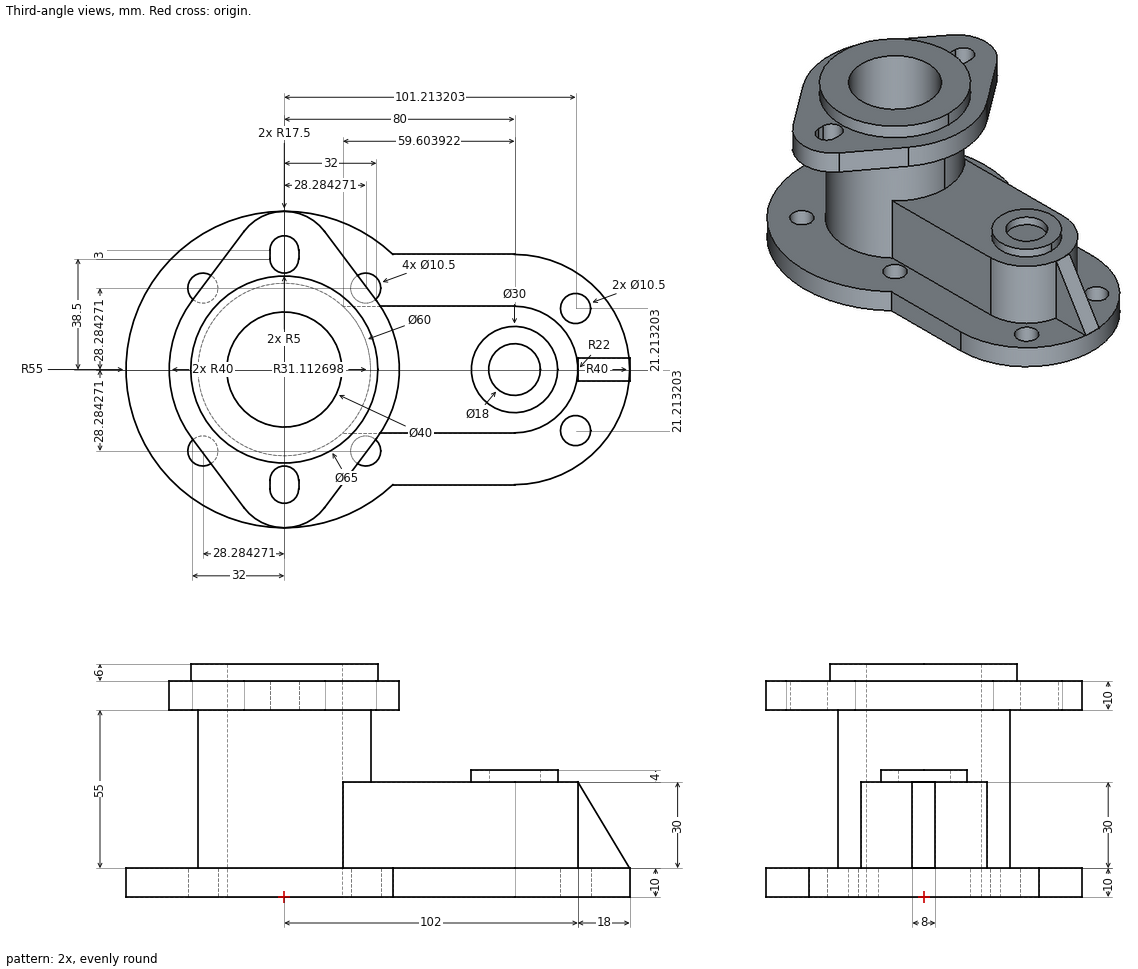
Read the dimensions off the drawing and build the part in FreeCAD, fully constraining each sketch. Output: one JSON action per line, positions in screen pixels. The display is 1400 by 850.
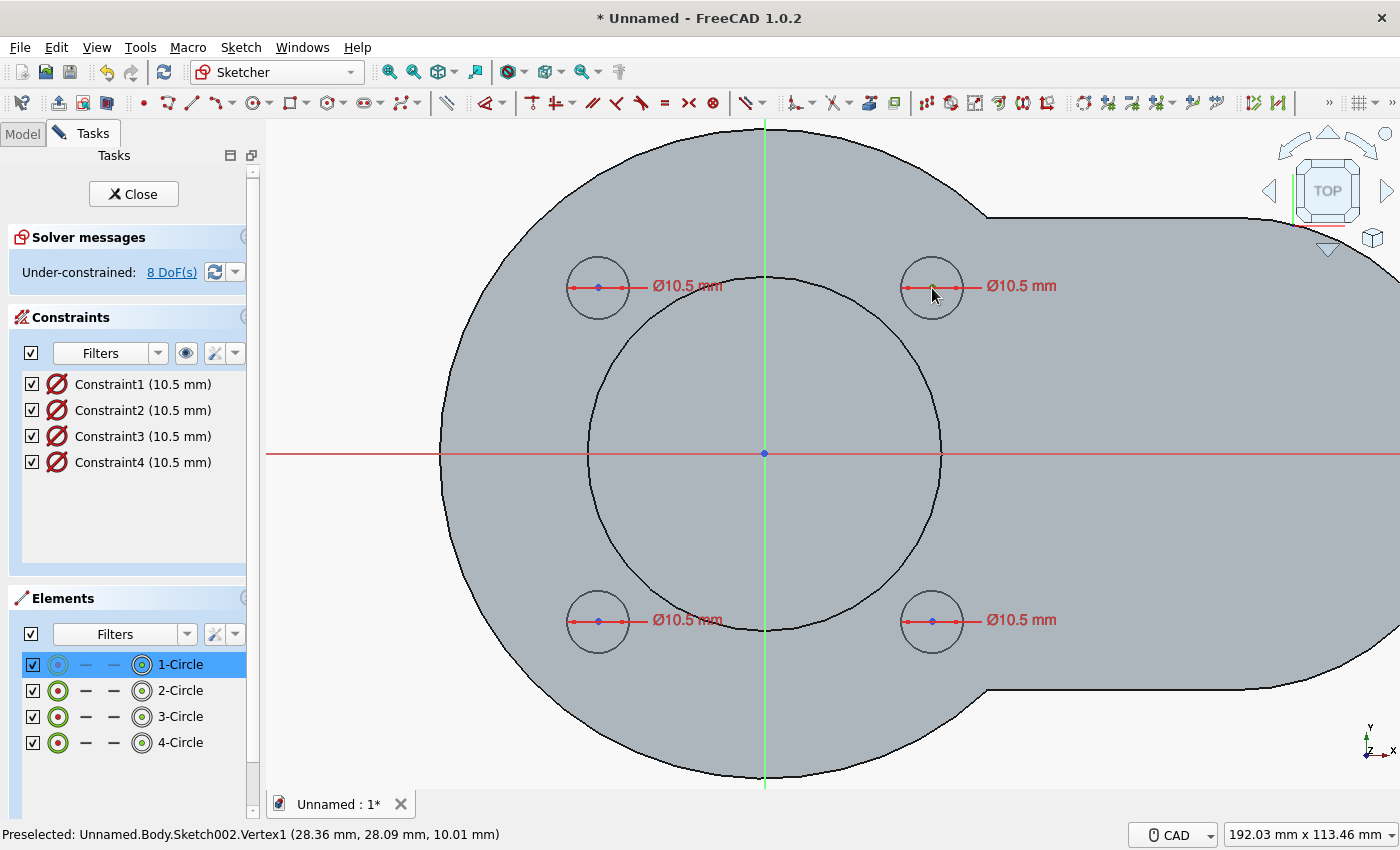
{"action": "left_click", "coordinate": [932, 622]}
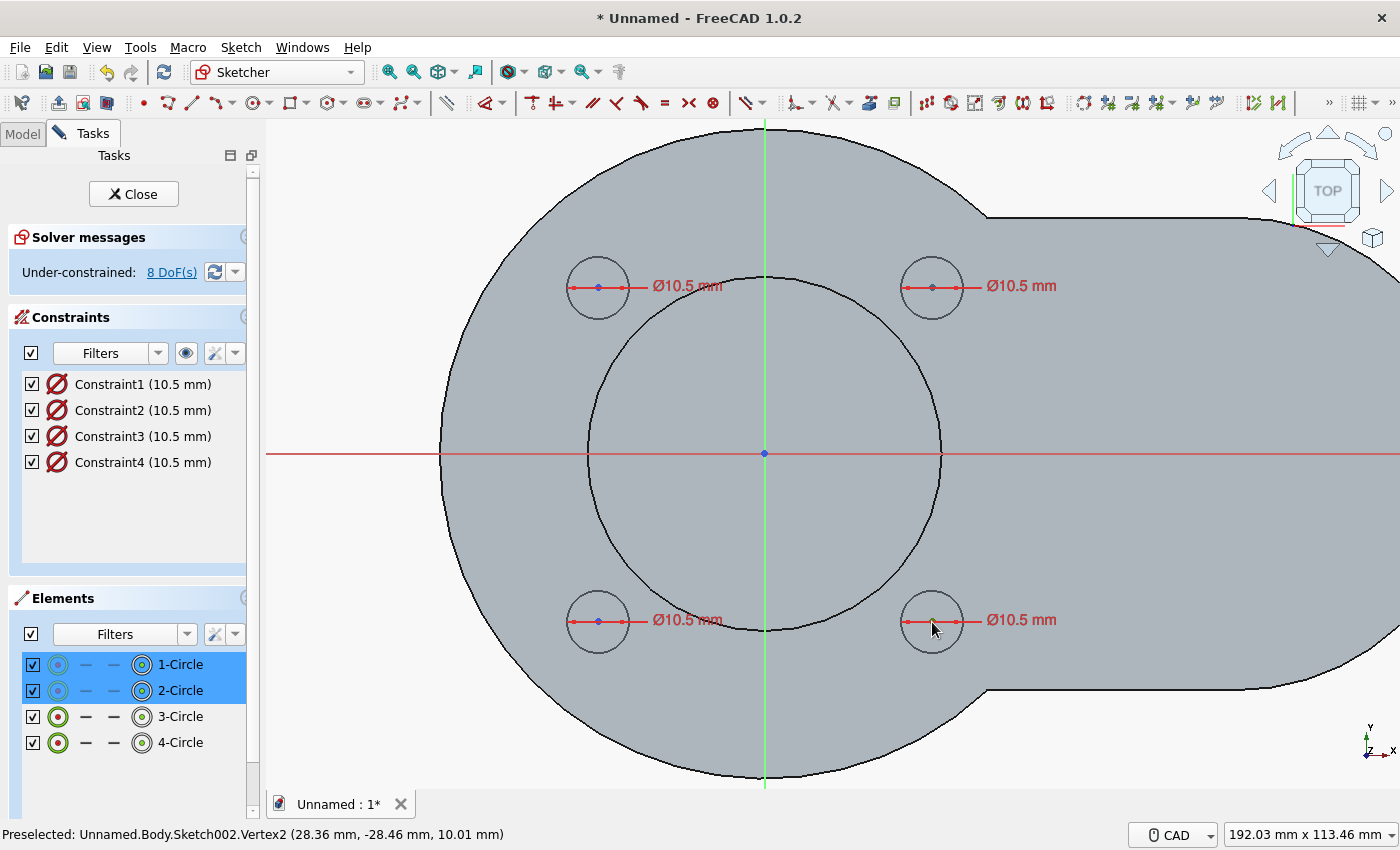
{"action": "key", "text": "v"}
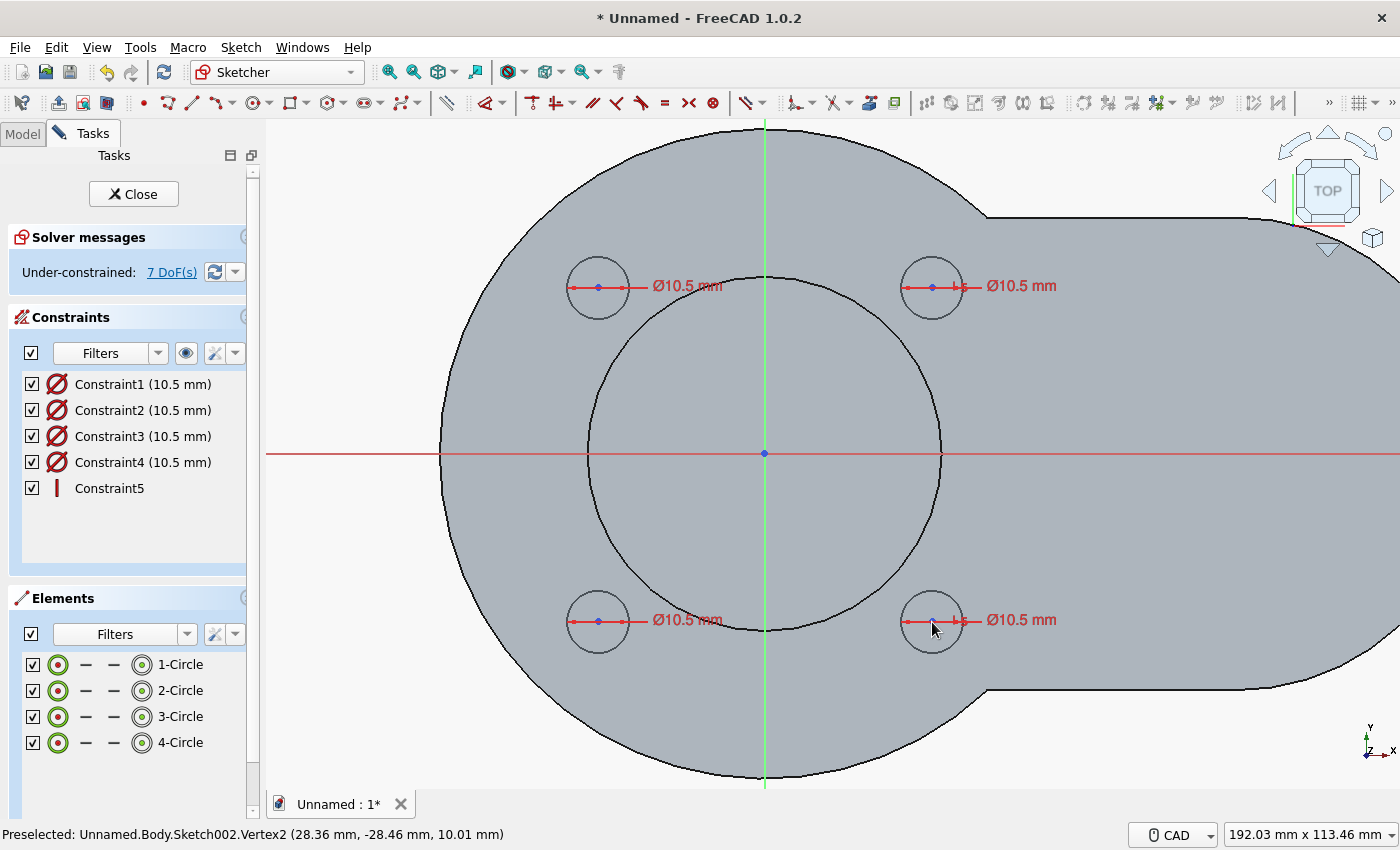
{"action": "left_click", "coordinate": [932, 622]}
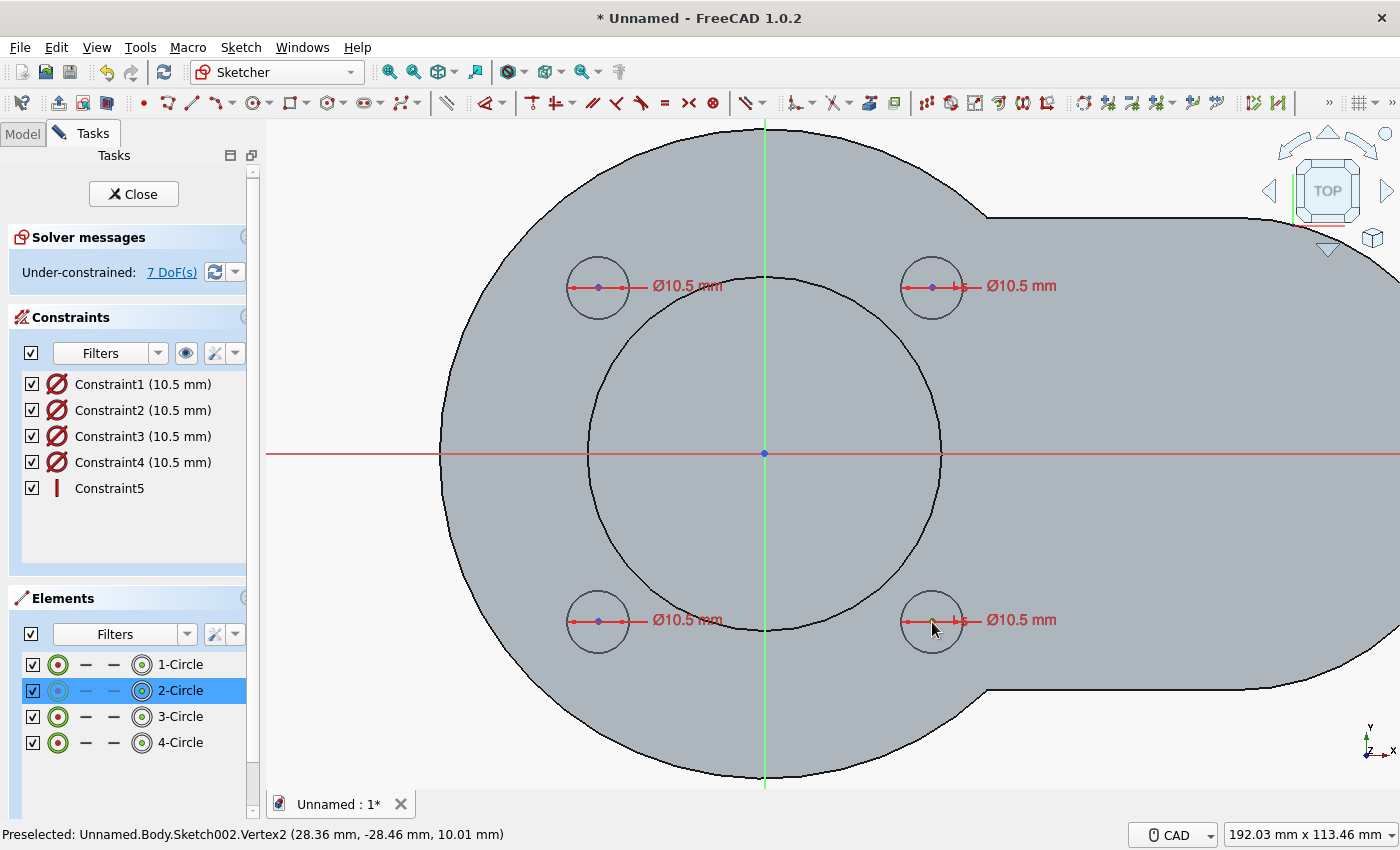
{"action": "left_click", "coordinate": [598, 622]}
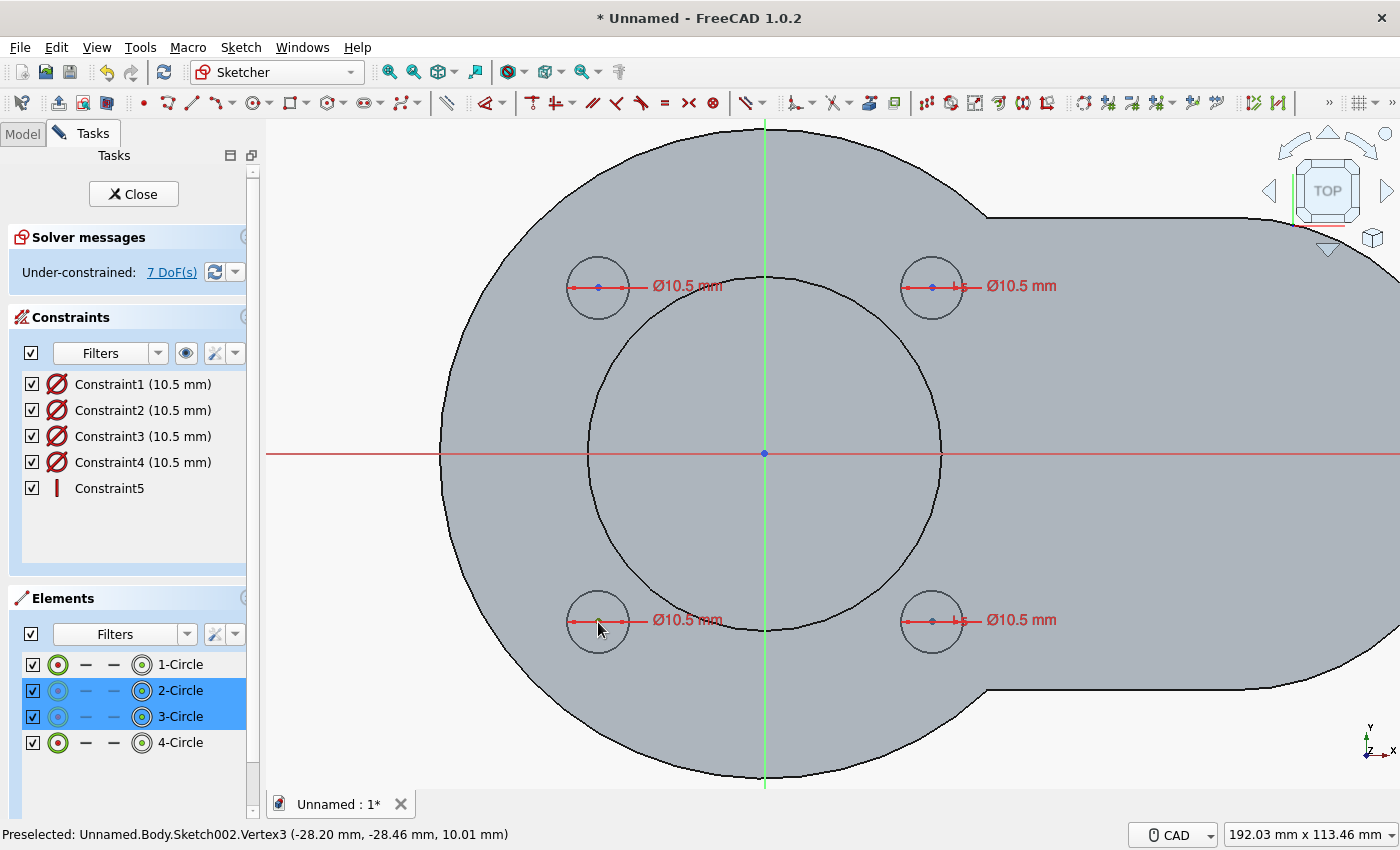
{"action": "key", "text": "h"}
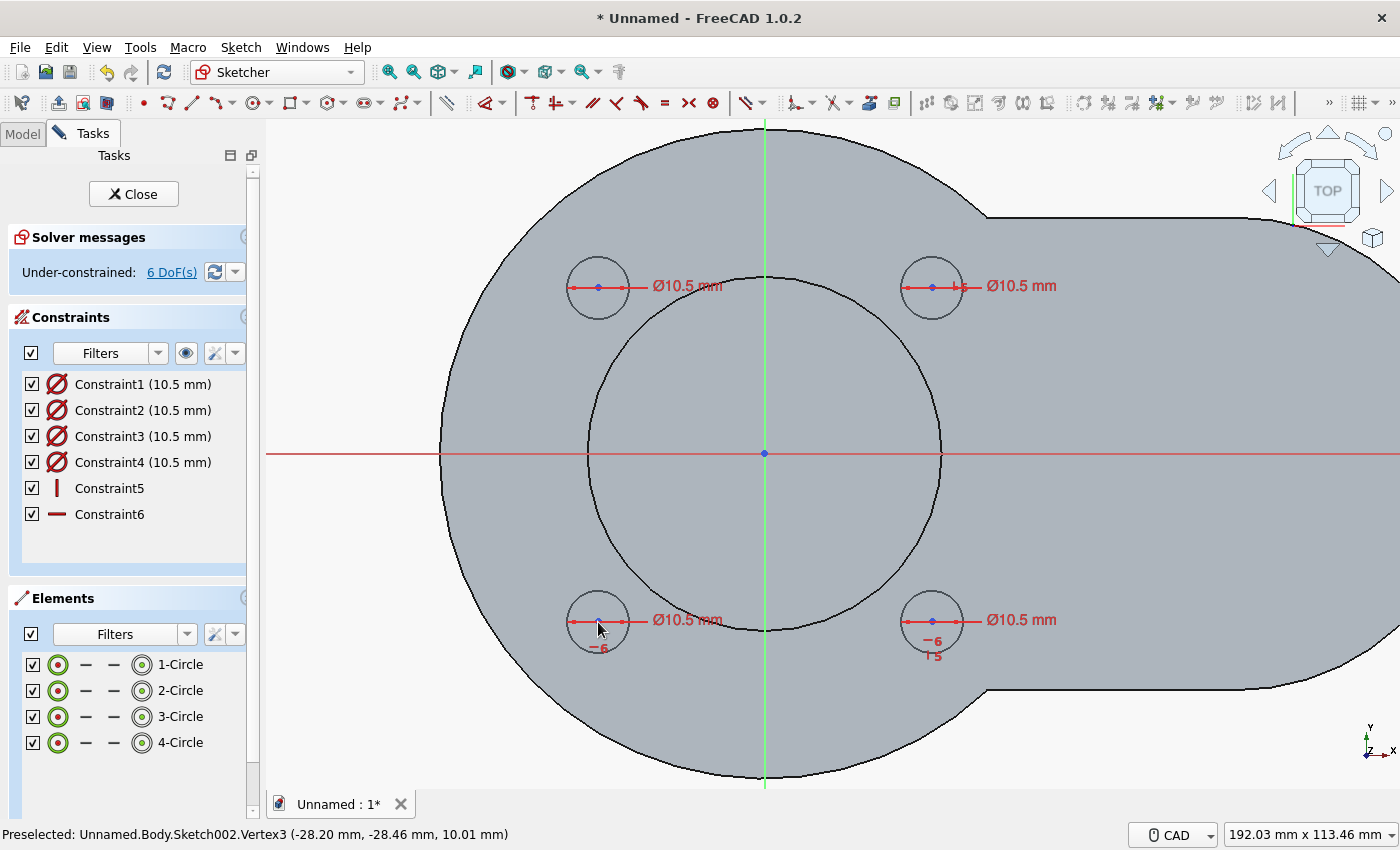
{"action": "left_click", "coordinate": [598, 622]}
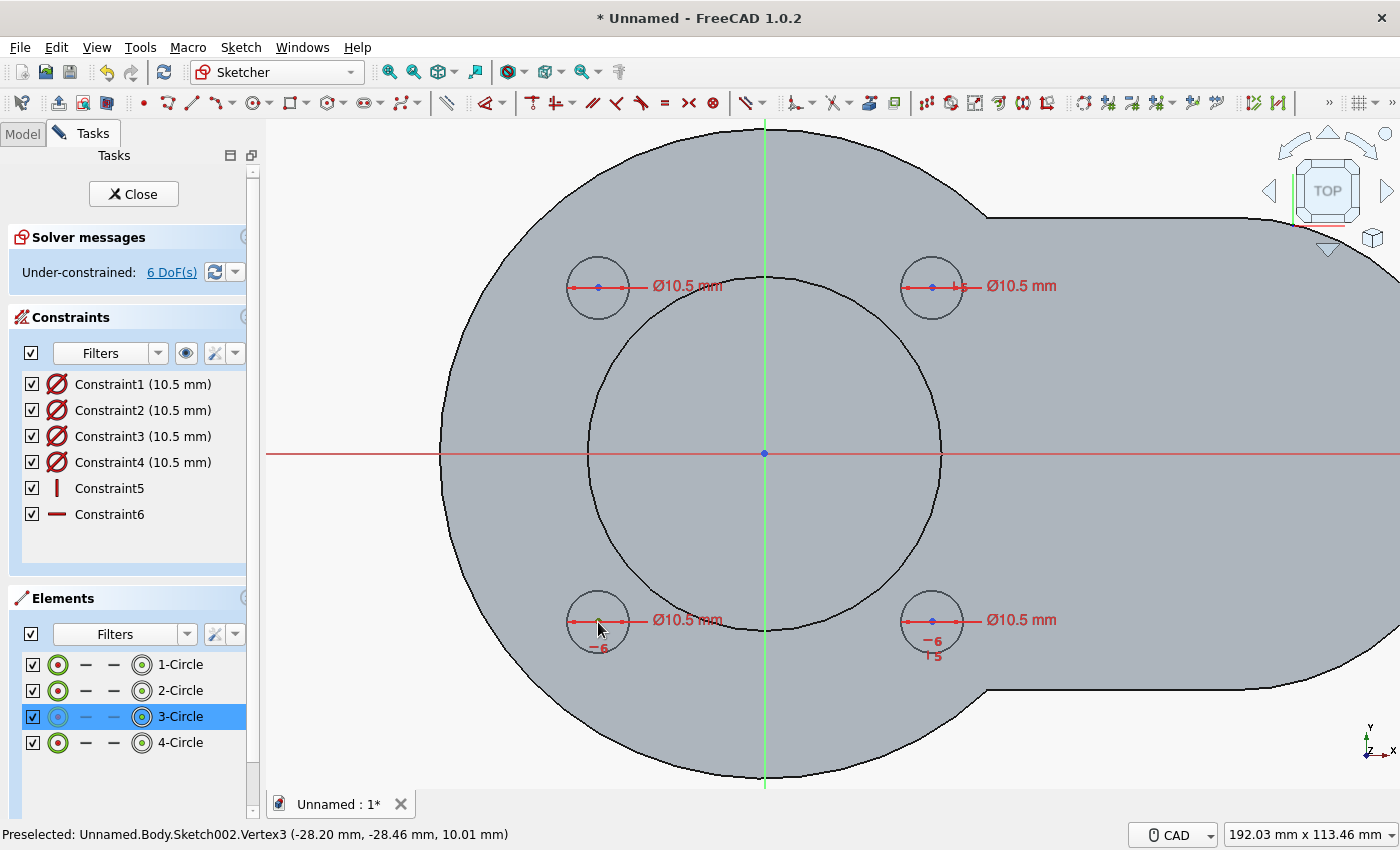
{"action": "left_click", "coordinate": [598, 288]}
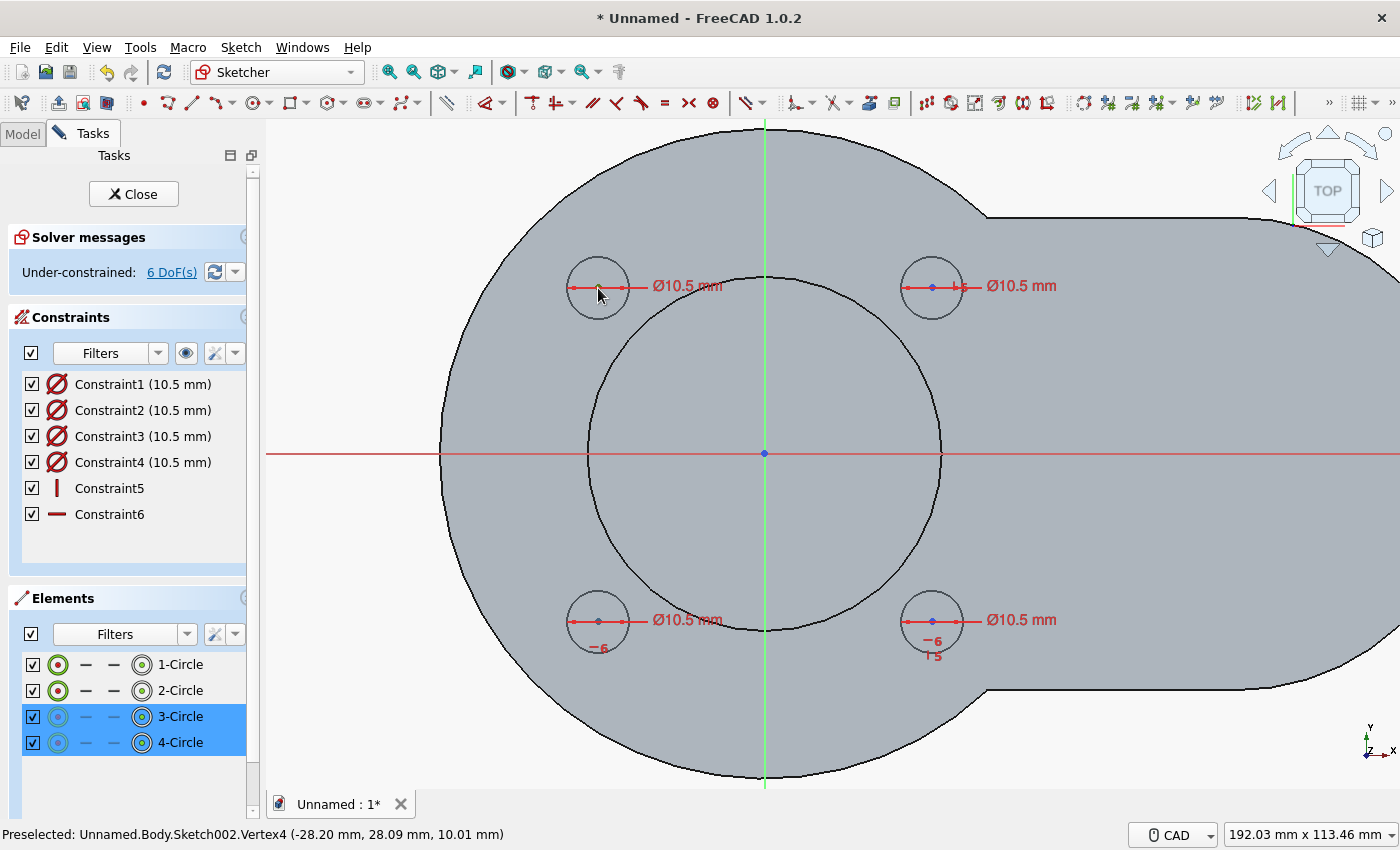
{"action": "left_click", "coordinate": [574, 104]}